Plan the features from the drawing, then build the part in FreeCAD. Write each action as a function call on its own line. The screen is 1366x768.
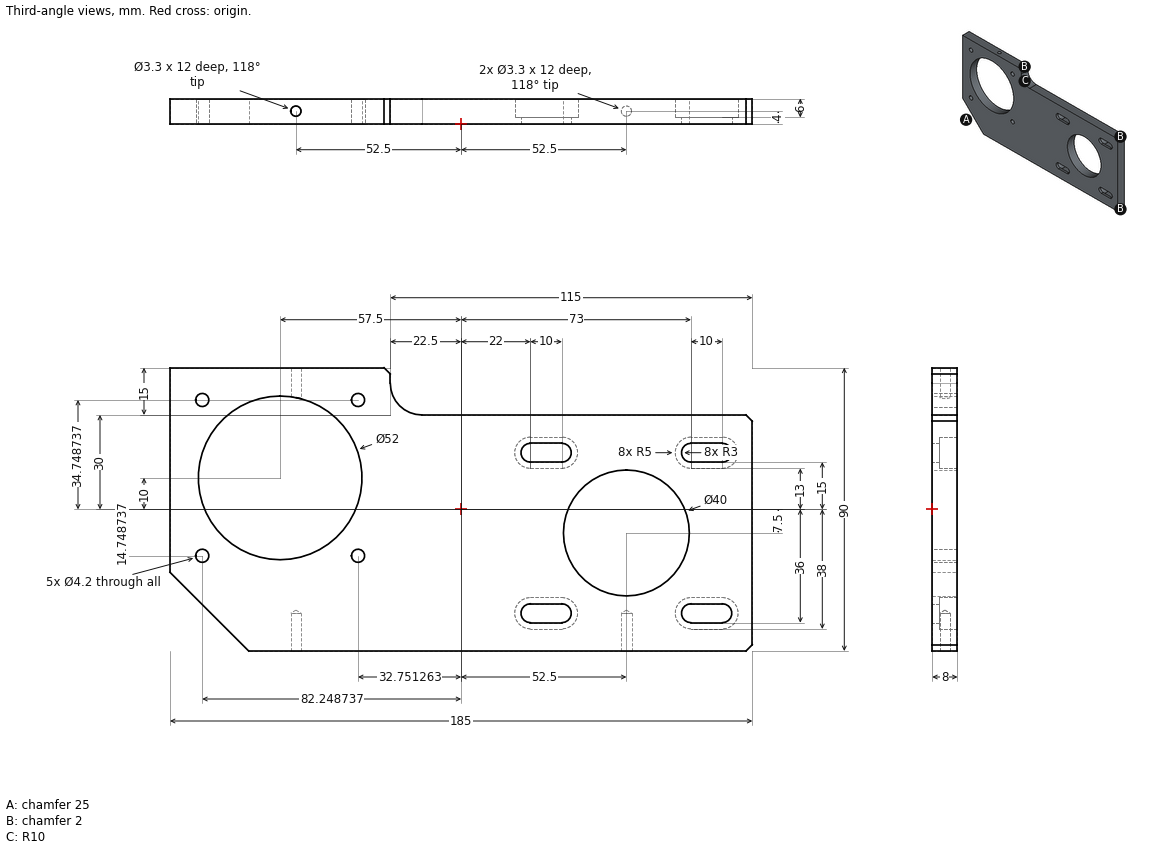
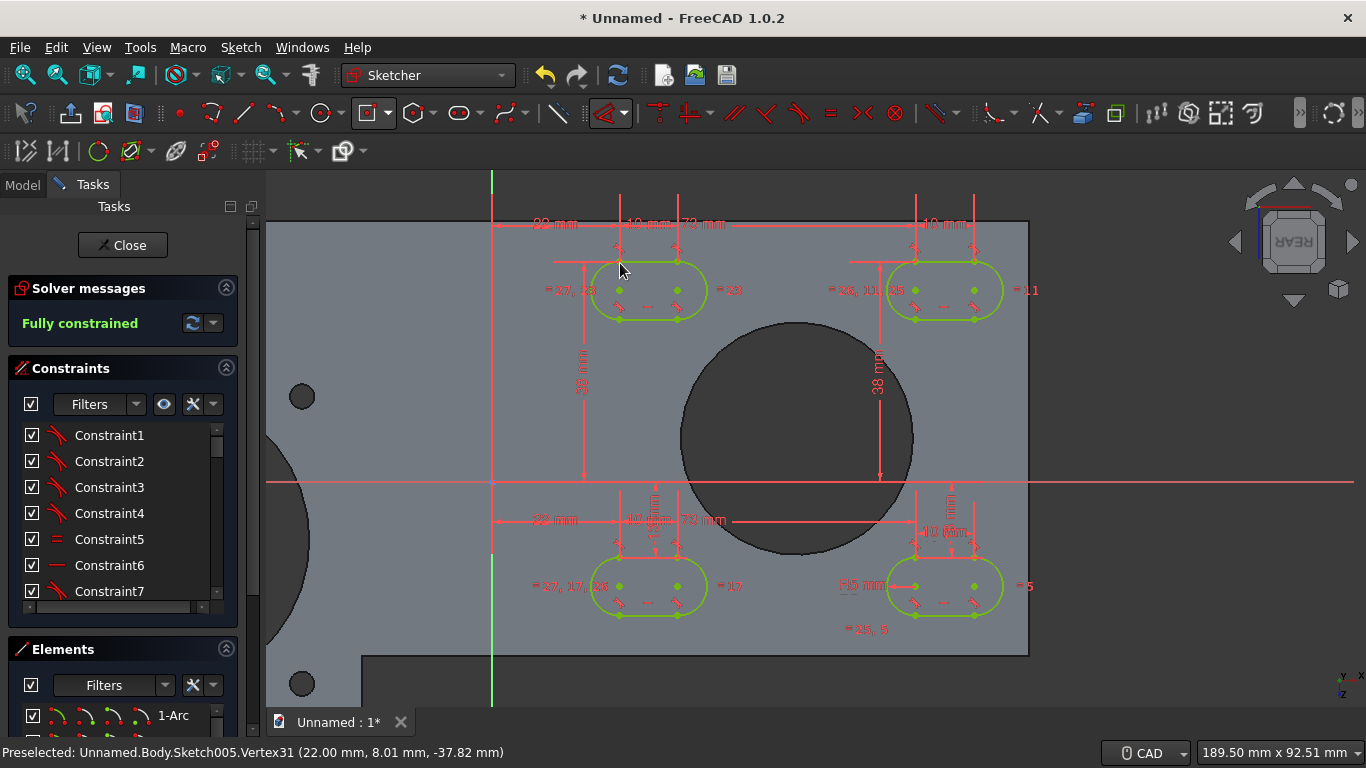
click(123, 245)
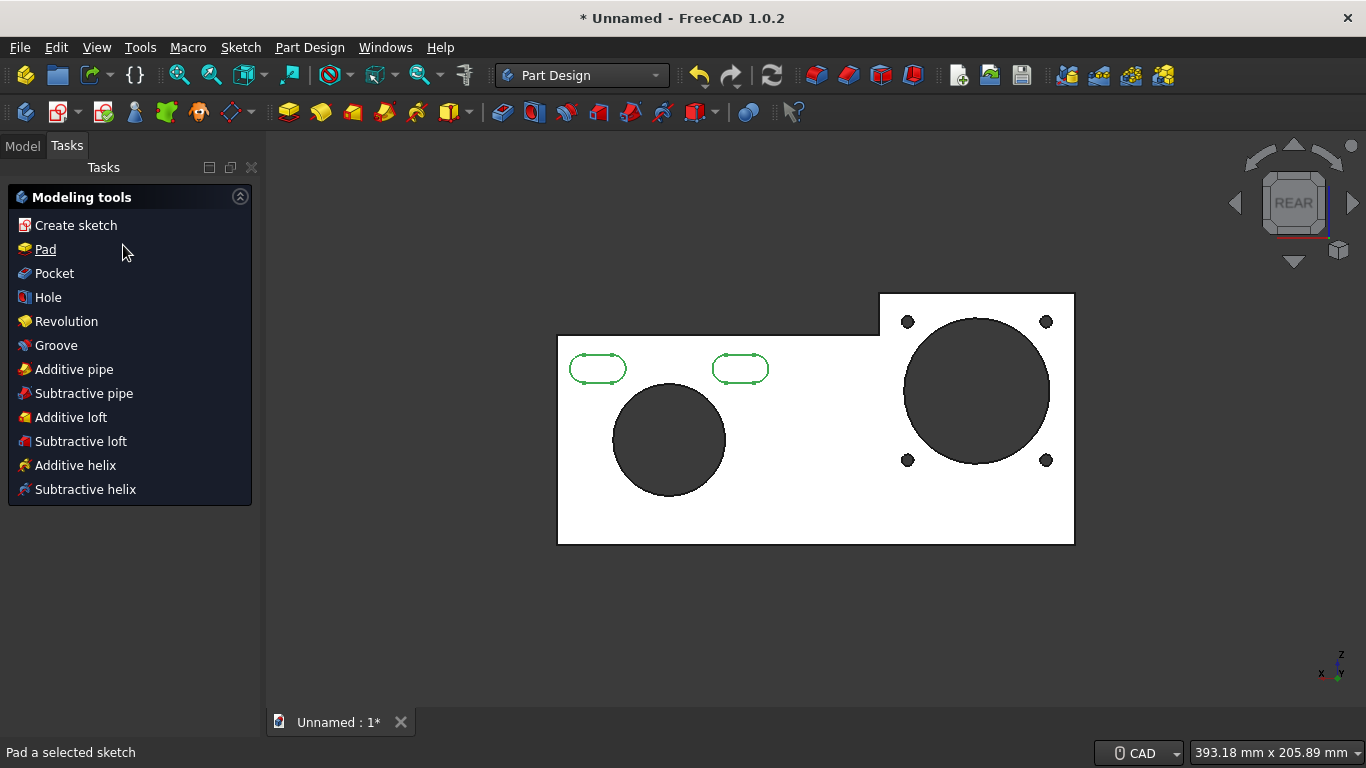
click(504, 112)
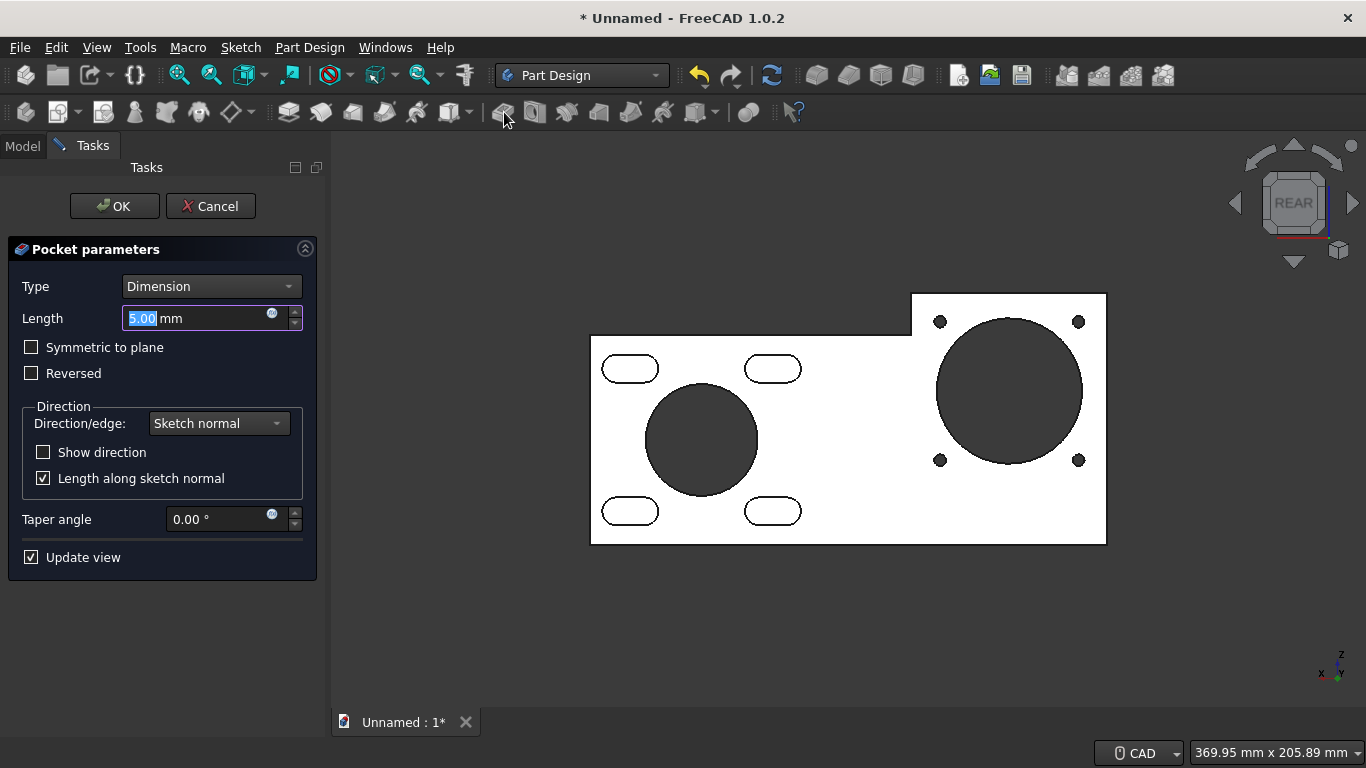
text(6)
key(Tab)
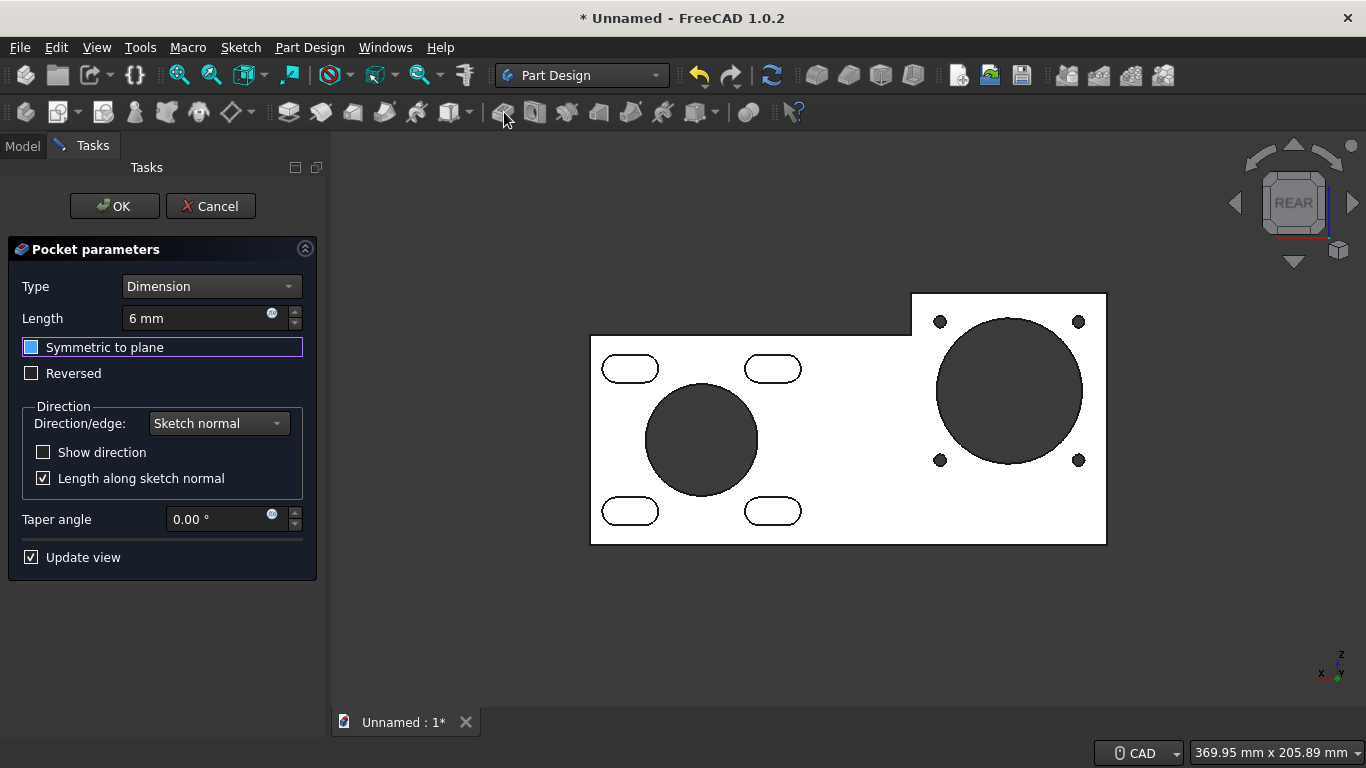
click(115, 206)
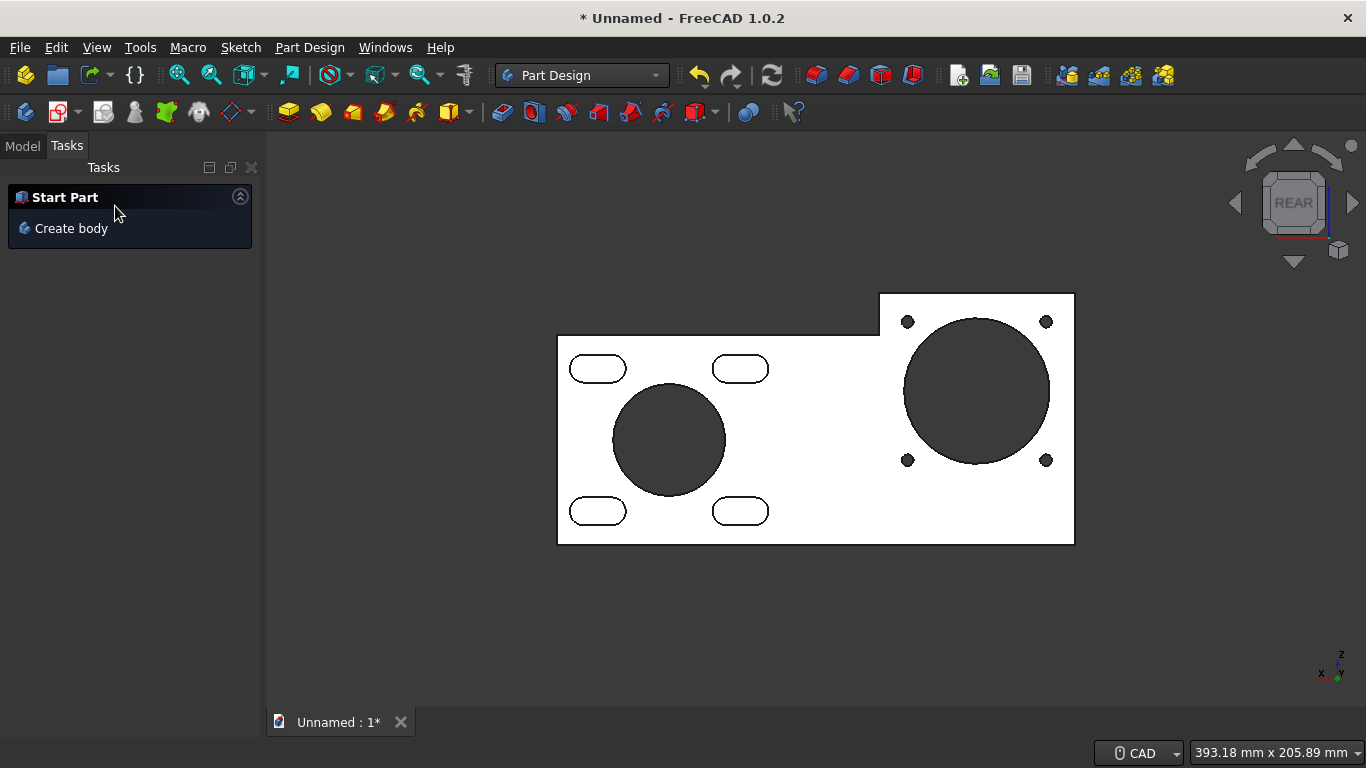
click(590, 510)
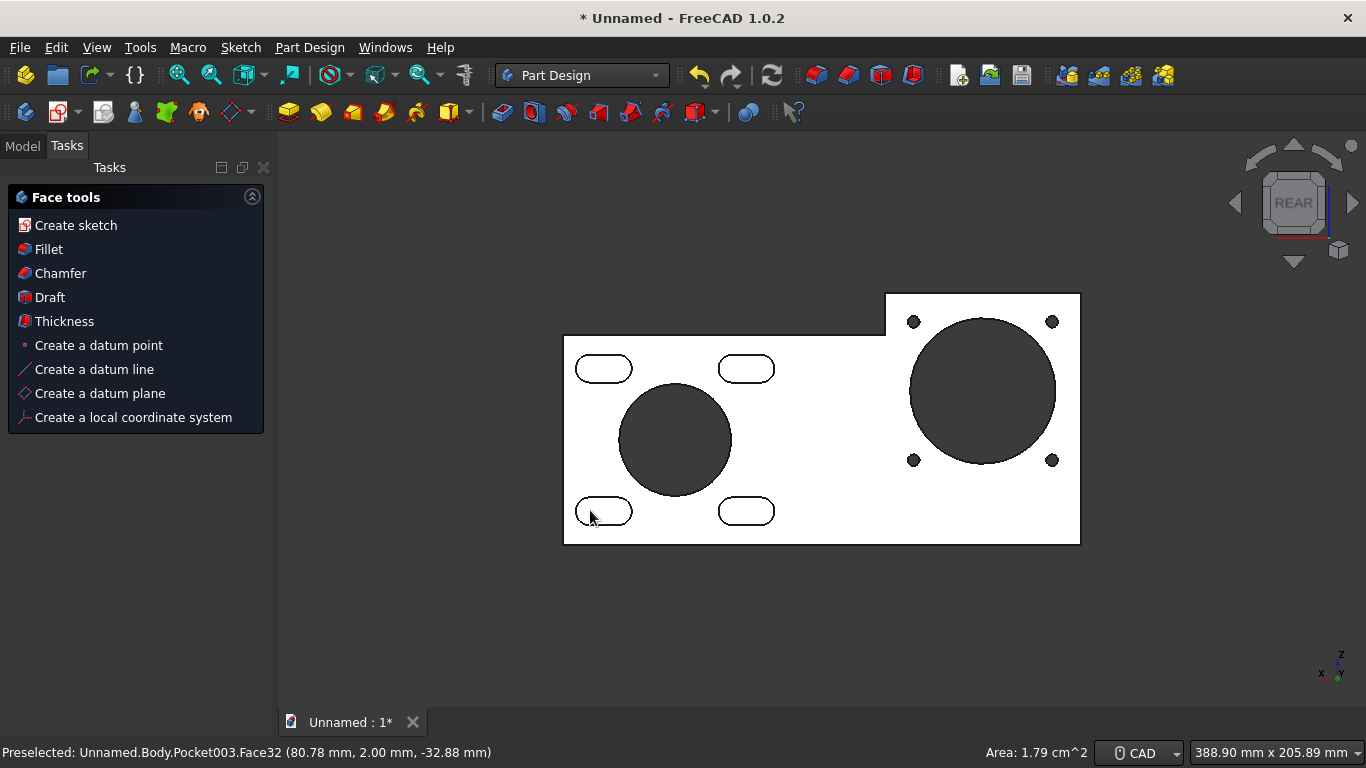
click(58, 112)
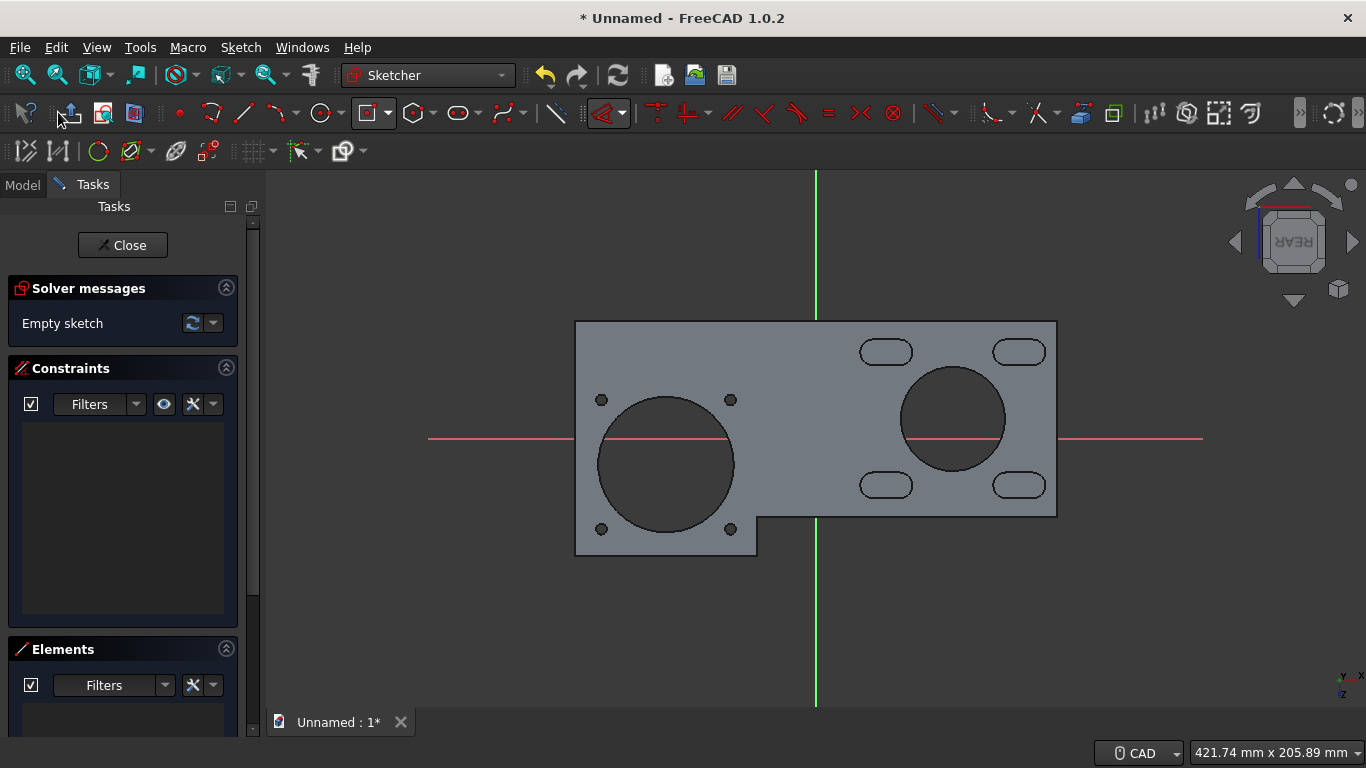
scroll(1076, 403, up, 4)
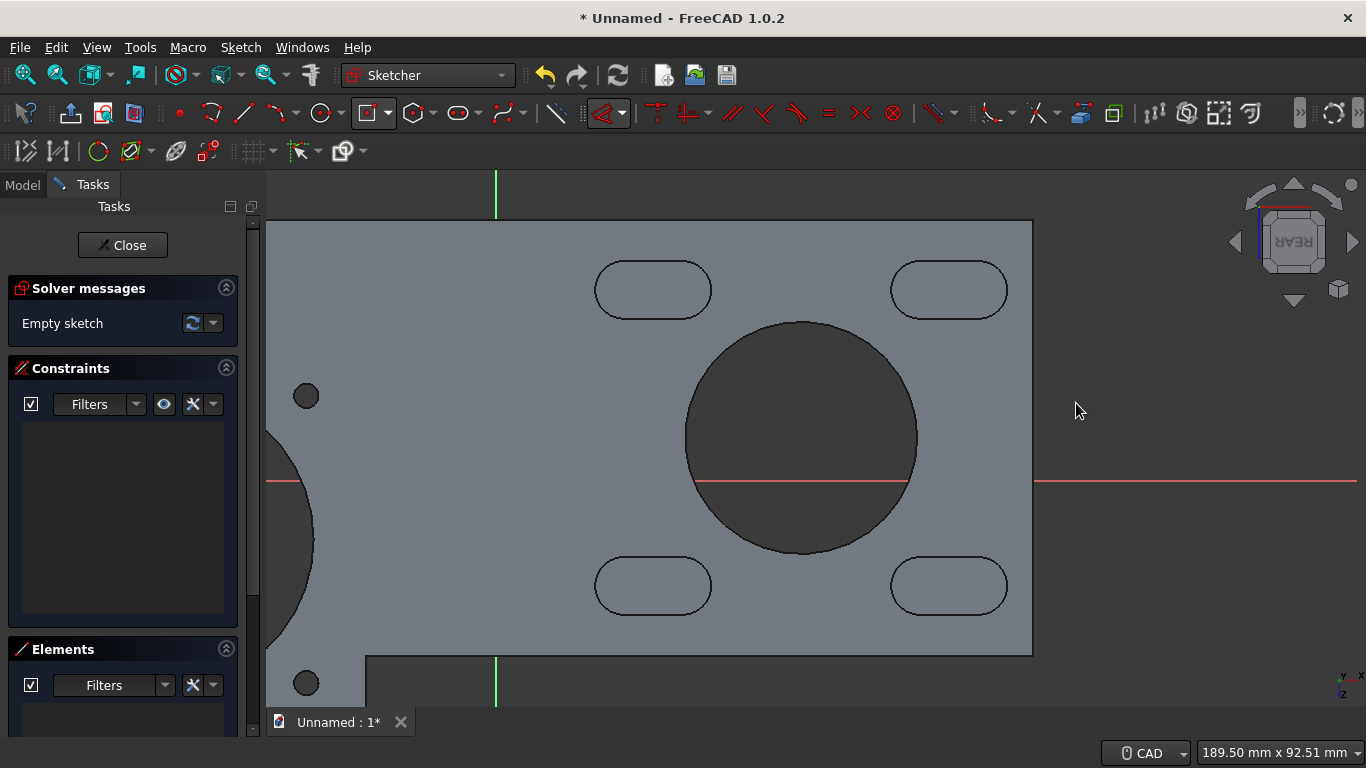
click(458, 114)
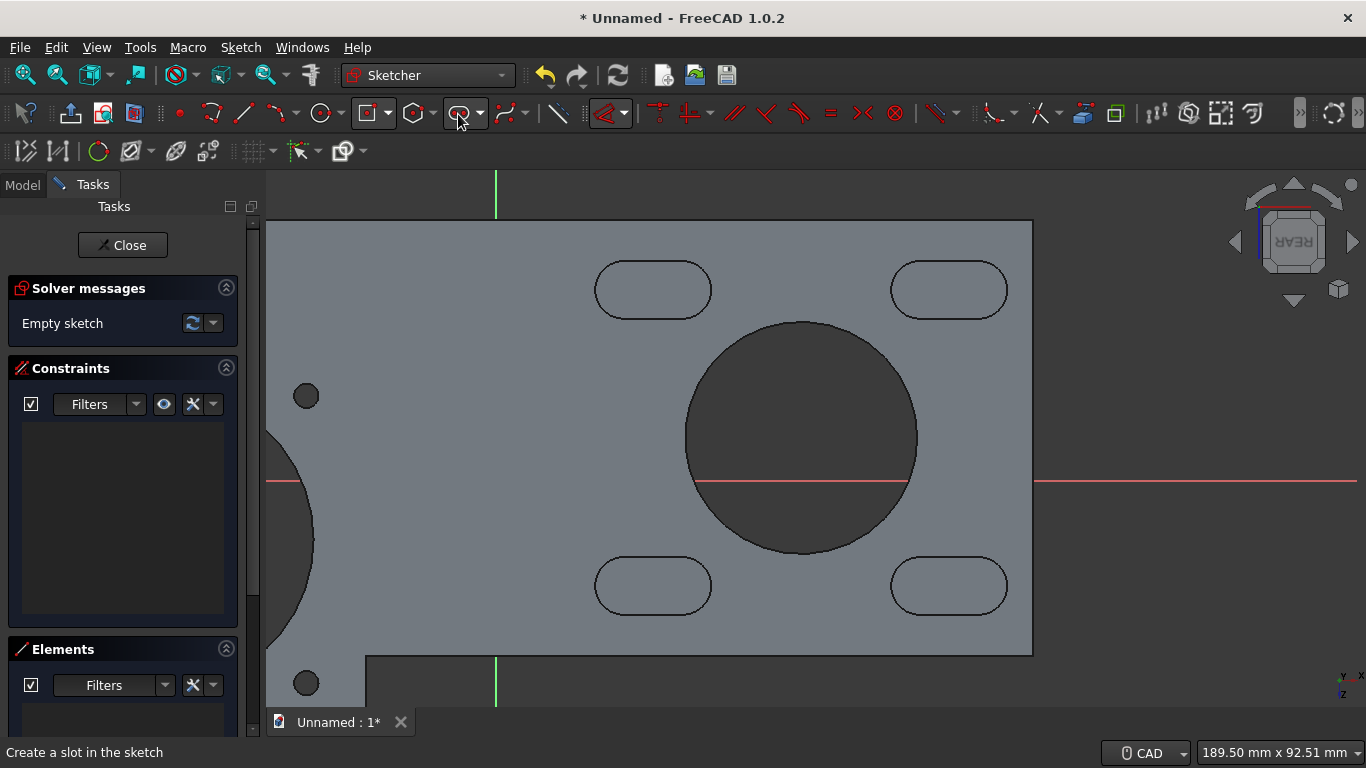
scroll(920, 586, up, 2)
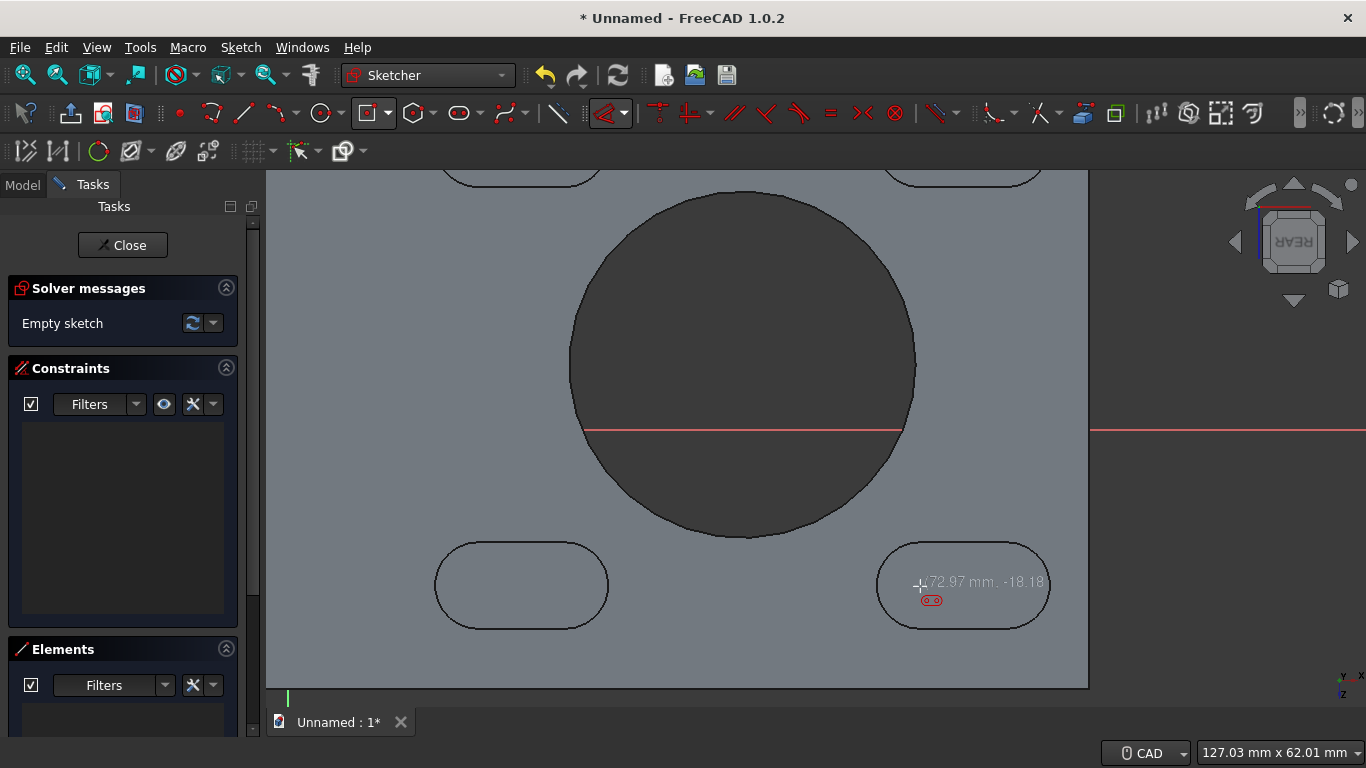
click(920, 586)